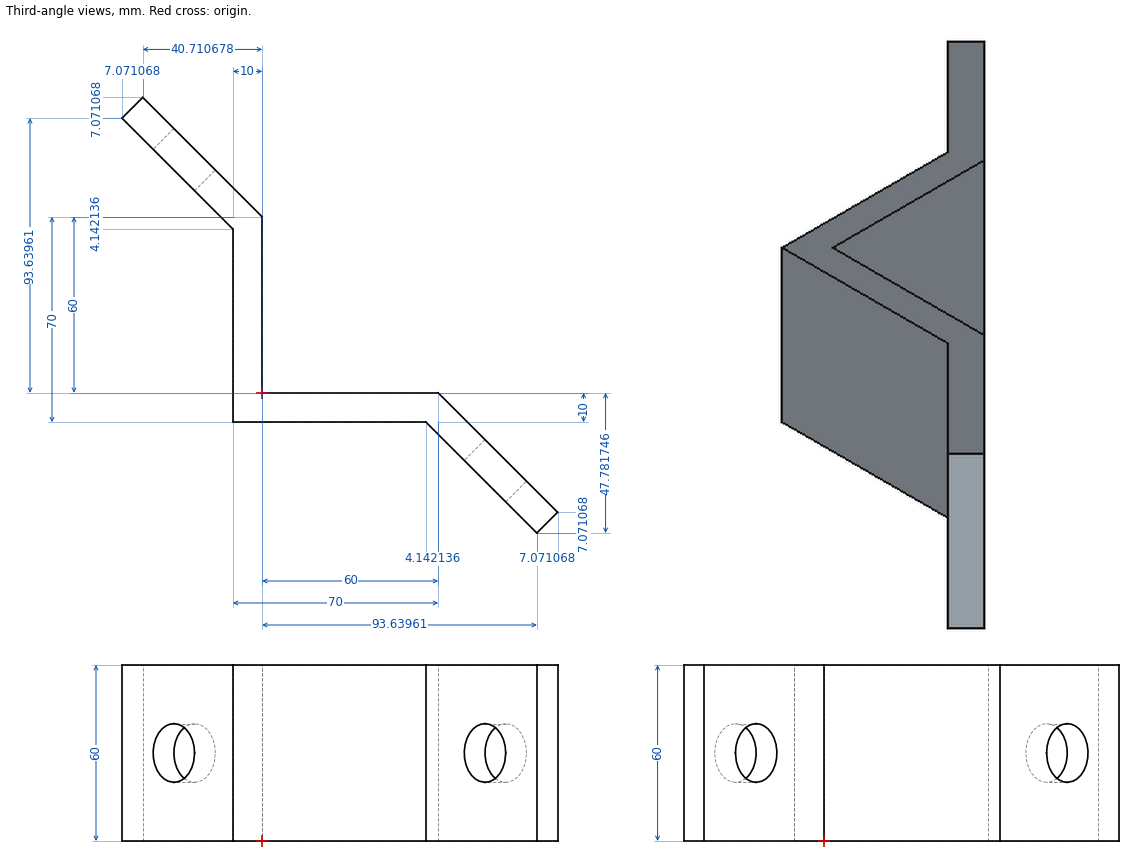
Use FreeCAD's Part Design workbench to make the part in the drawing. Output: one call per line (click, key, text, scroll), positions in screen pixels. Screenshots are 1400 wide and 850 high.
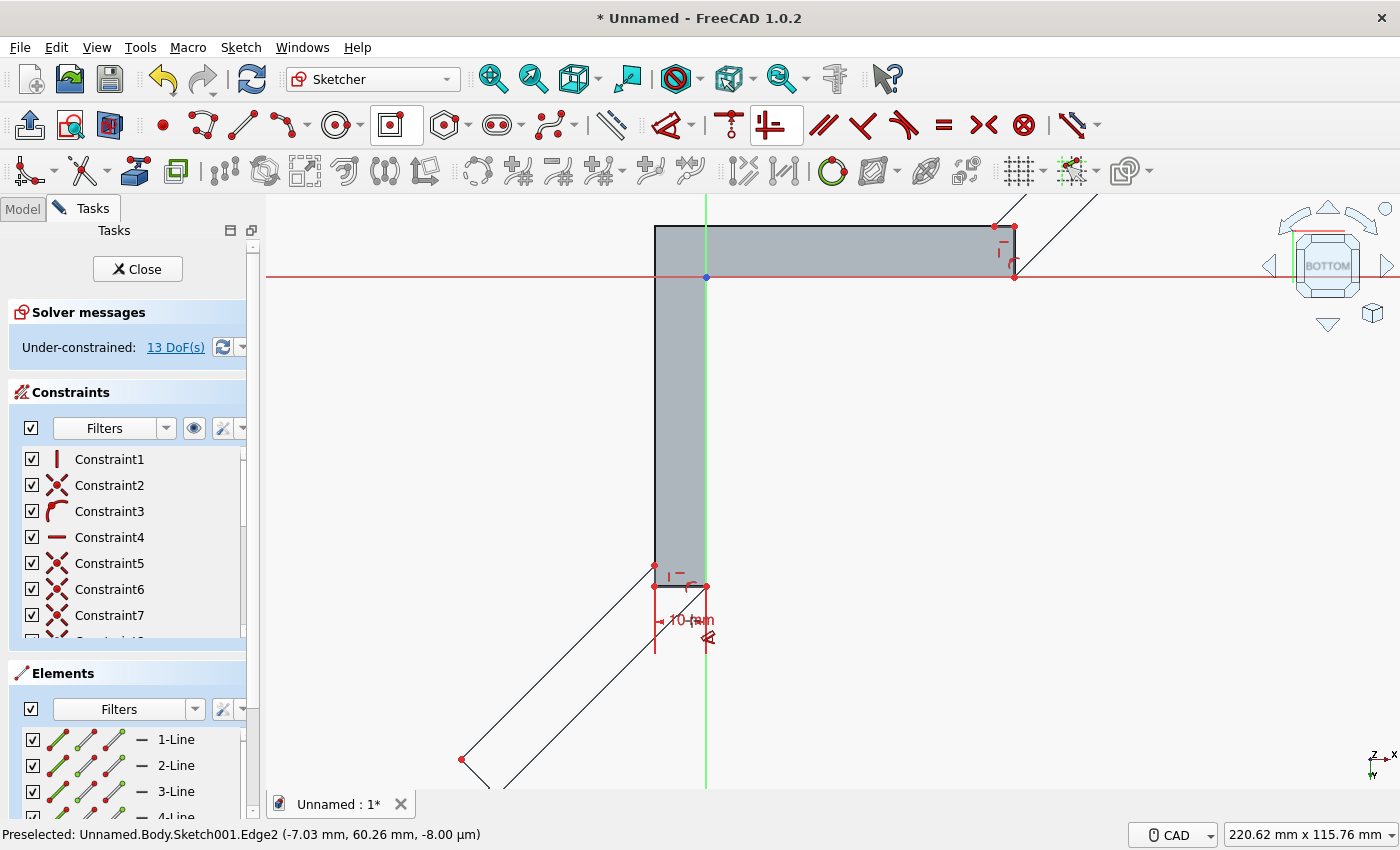
scroll(1014, 262, up, 2)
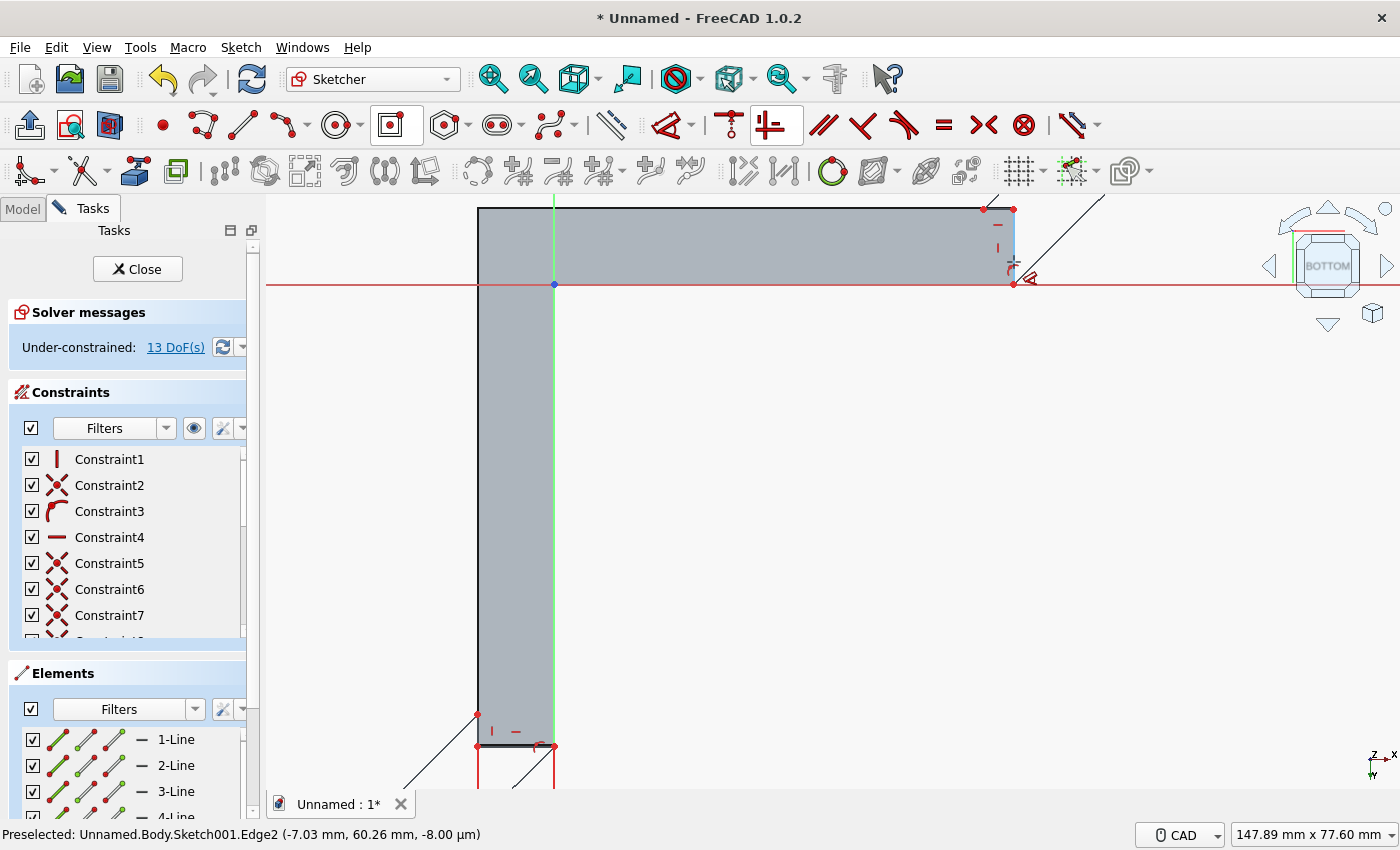
click(1014, 262)
click(1048, 231)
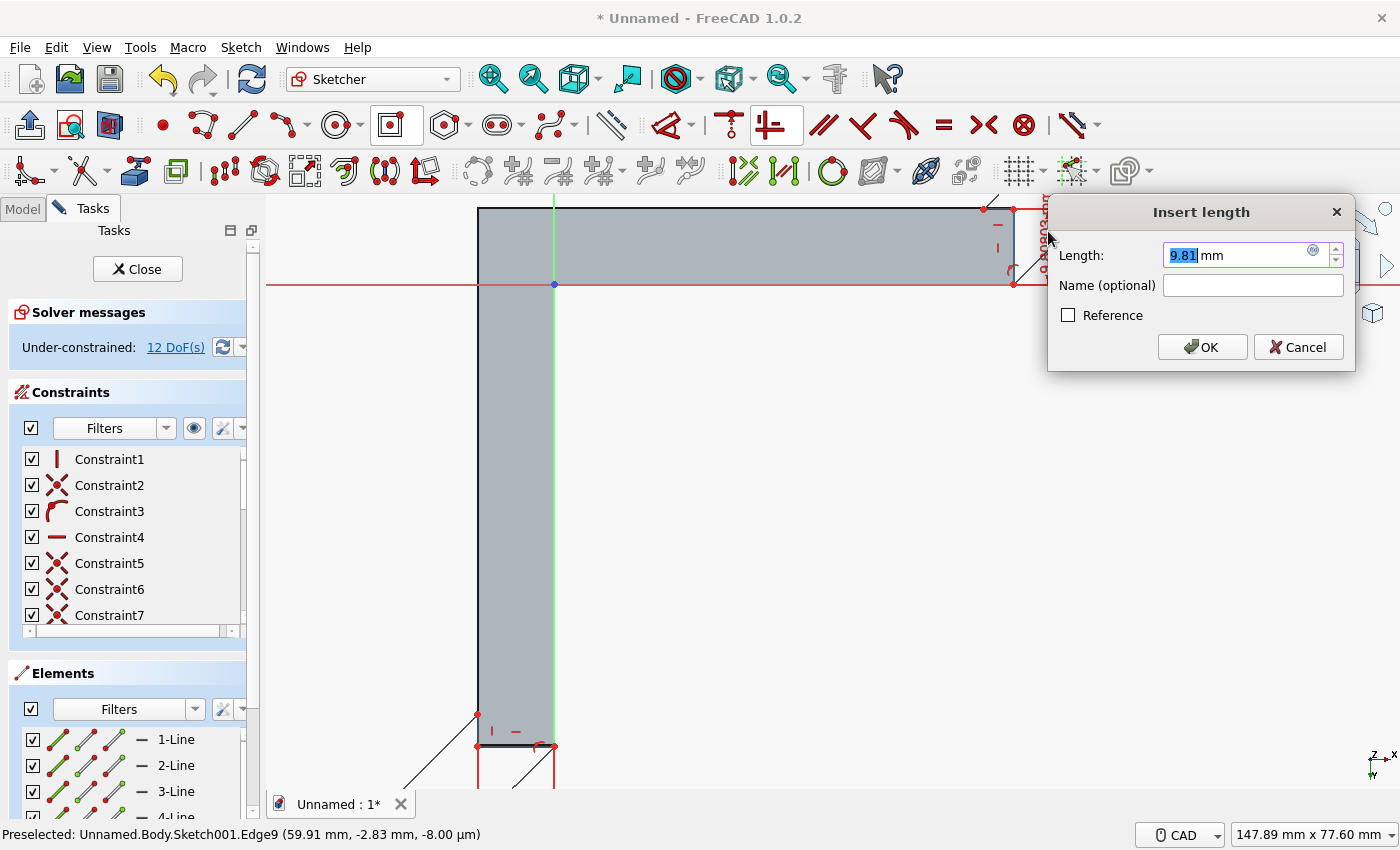
text(10)
key(Return)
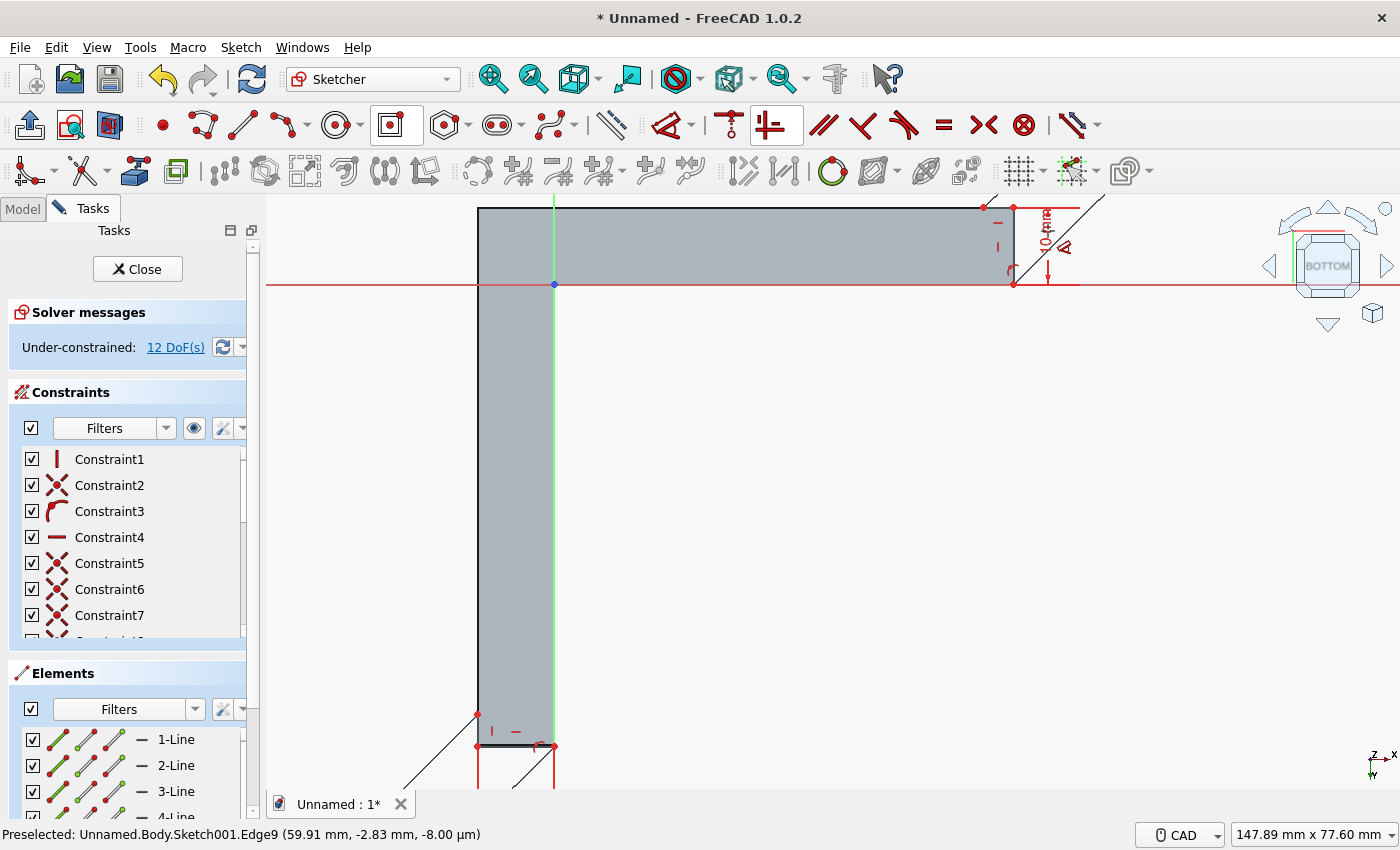
click(478, 747)
click(444, 516)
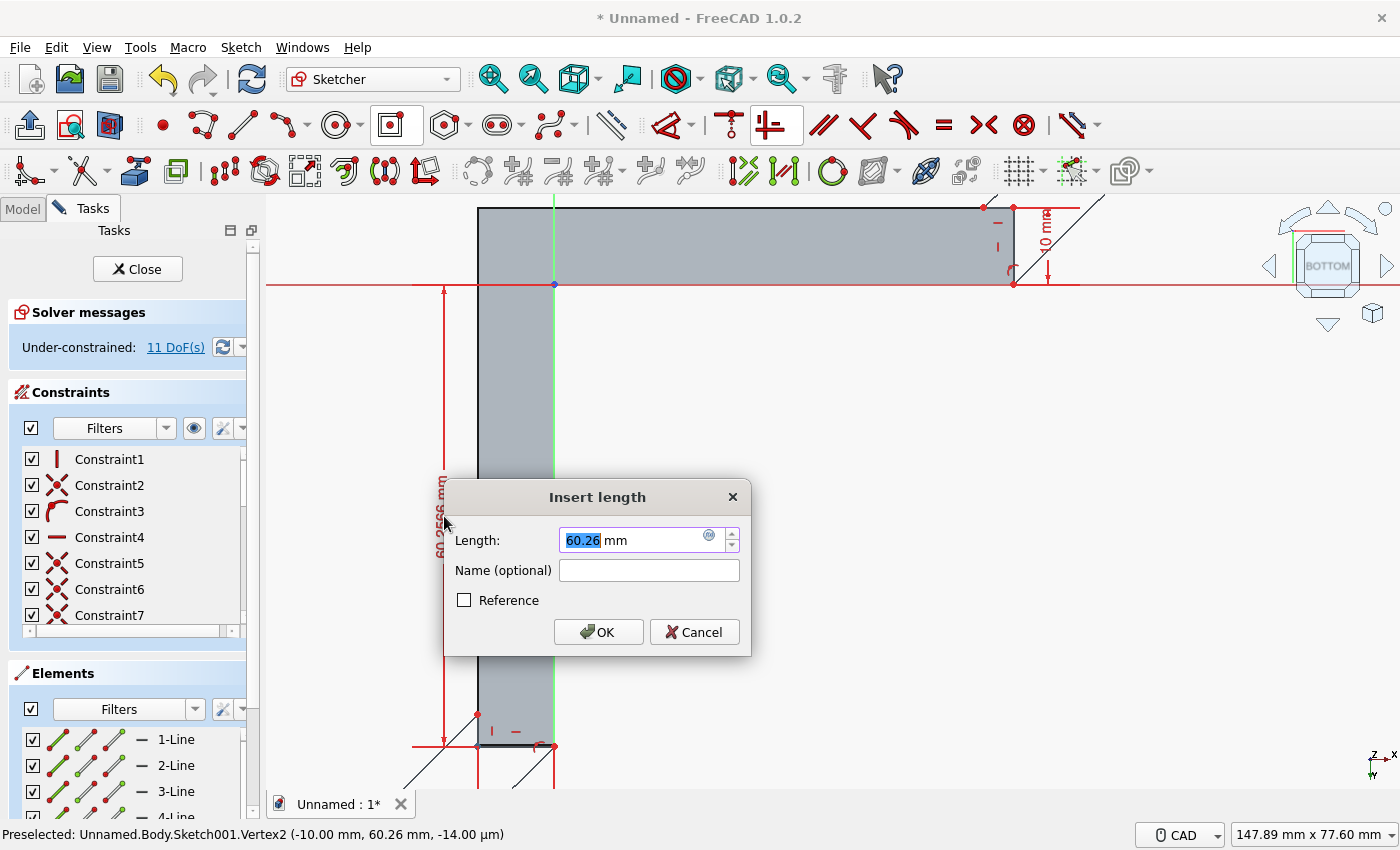
text(60)
key(Return)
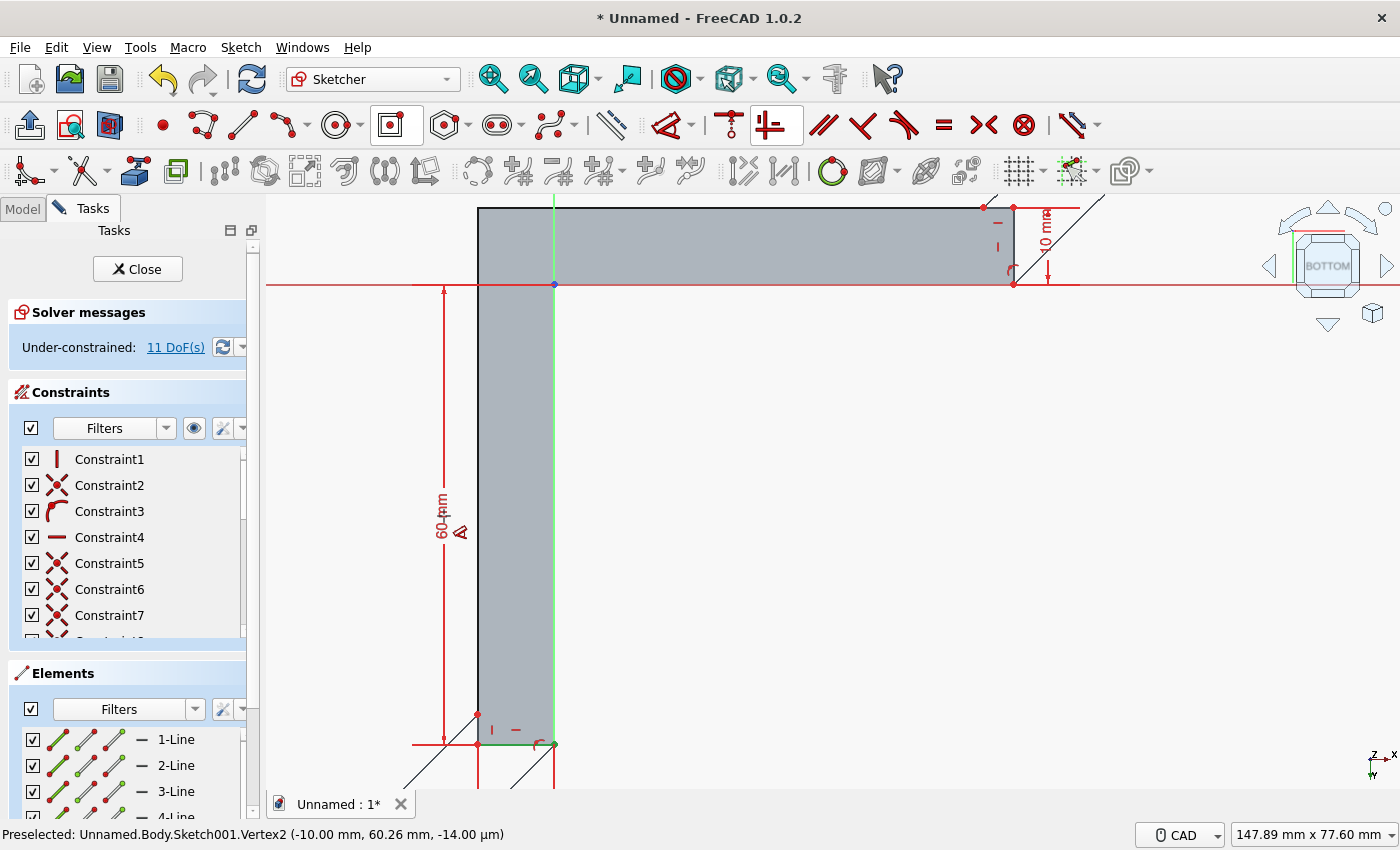
click(1014, 285)
click(784, 251)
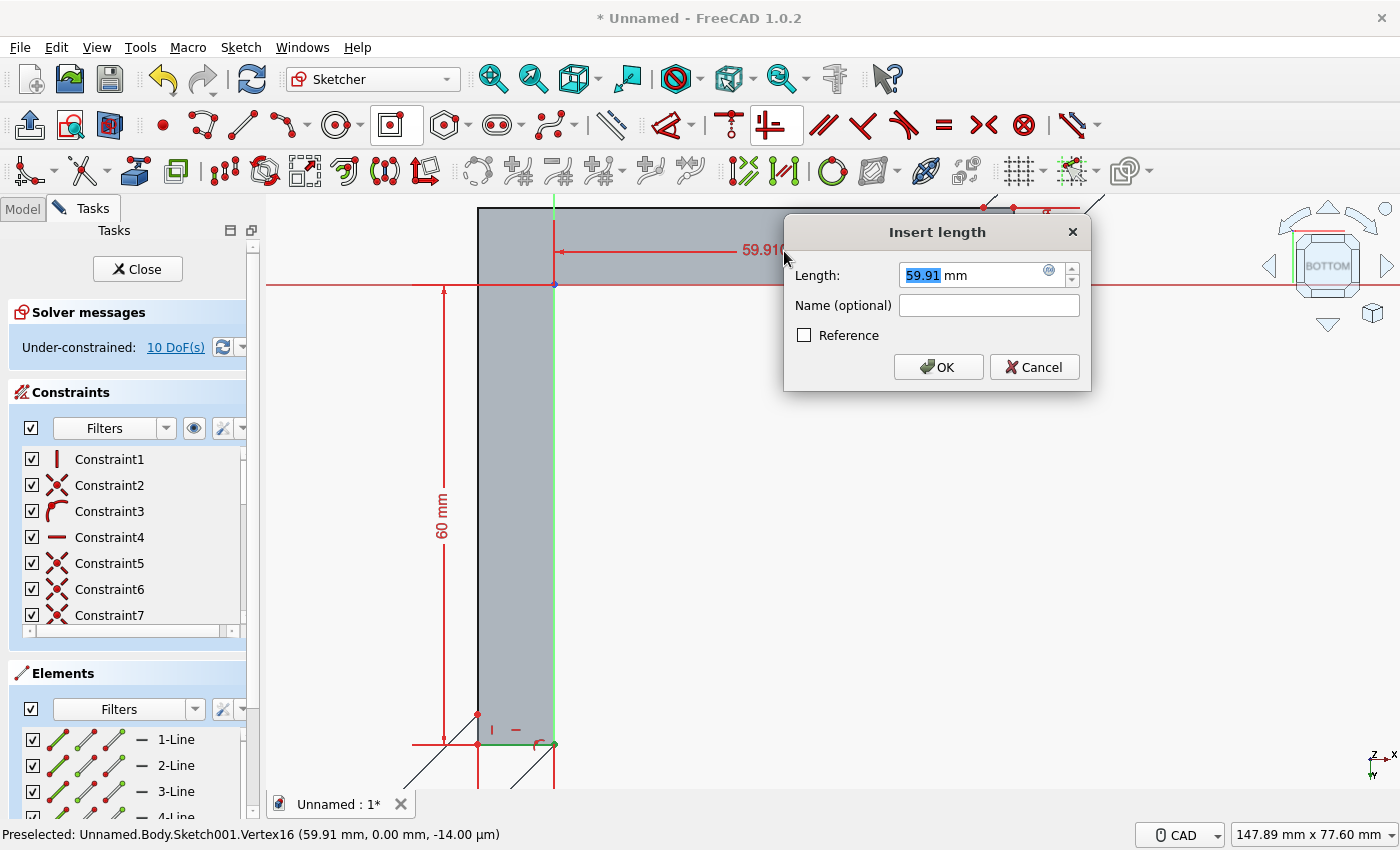
text(60)
key(Return)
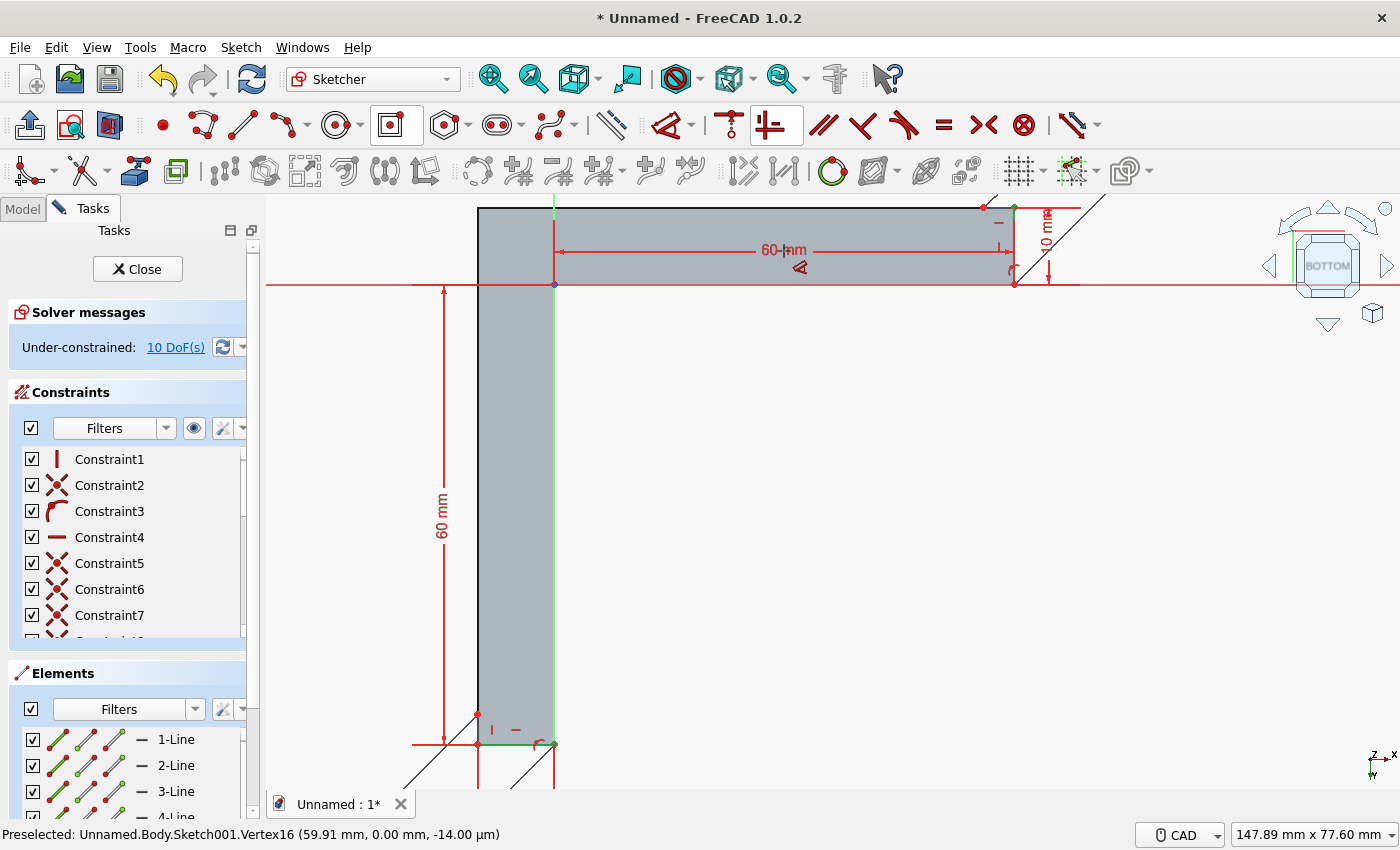
scroll(478, 736, up, 3)